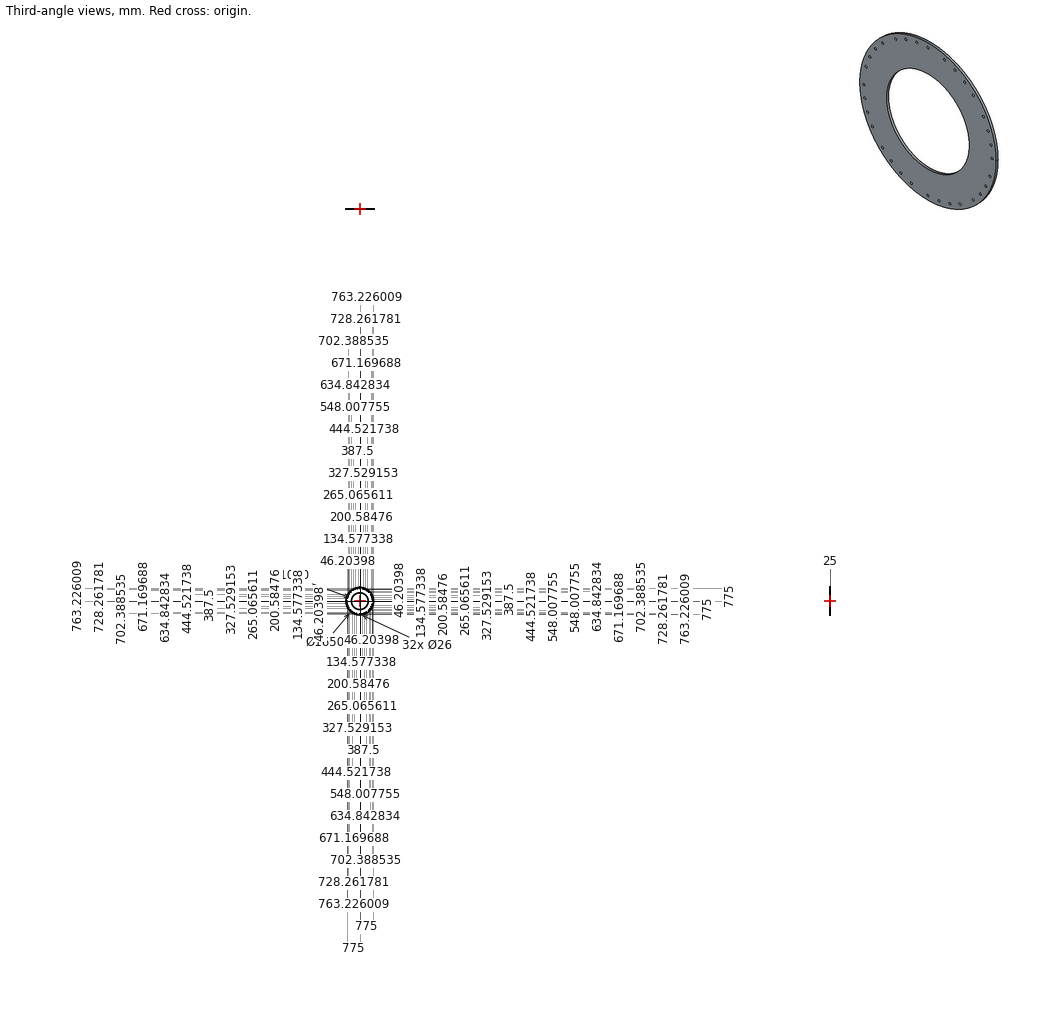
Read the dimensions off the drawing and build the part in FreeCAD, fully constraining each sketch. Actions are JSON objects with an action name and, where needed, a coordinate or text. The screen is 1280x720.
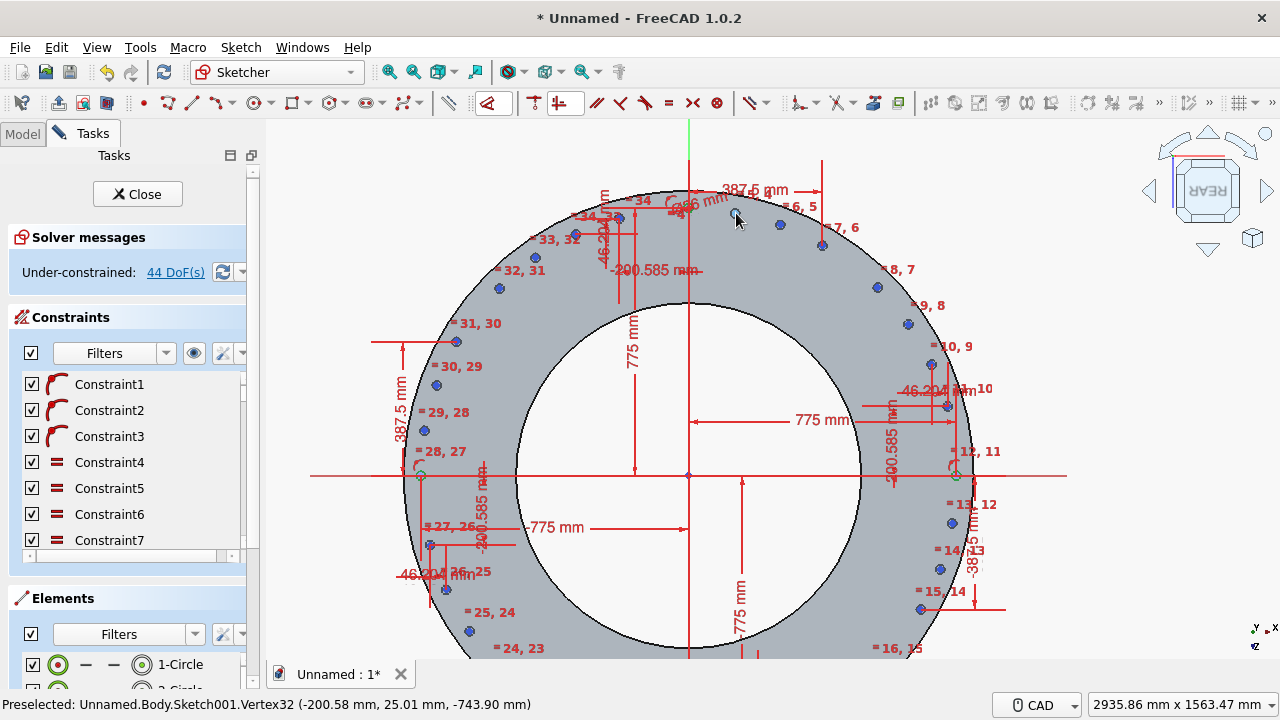
{"action": "left_click", "coordinate": [735, 213]}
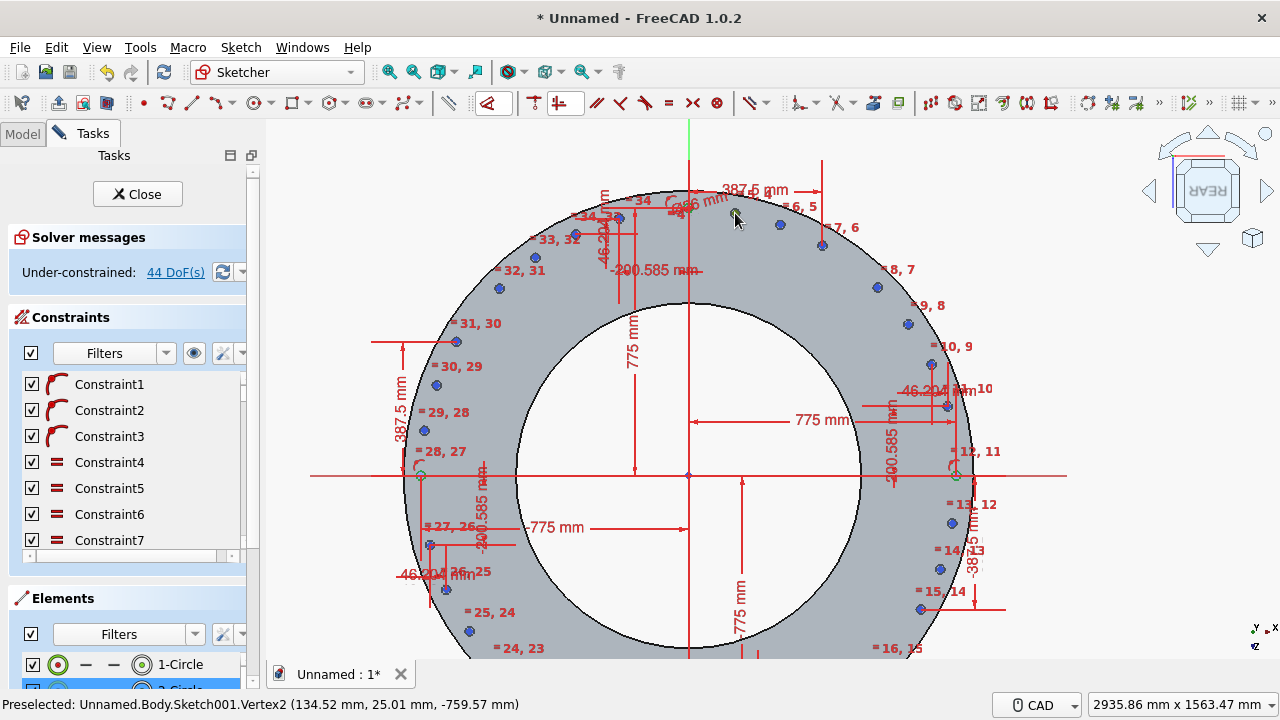
{"action": "left_click", "coordinate": [506, 104]}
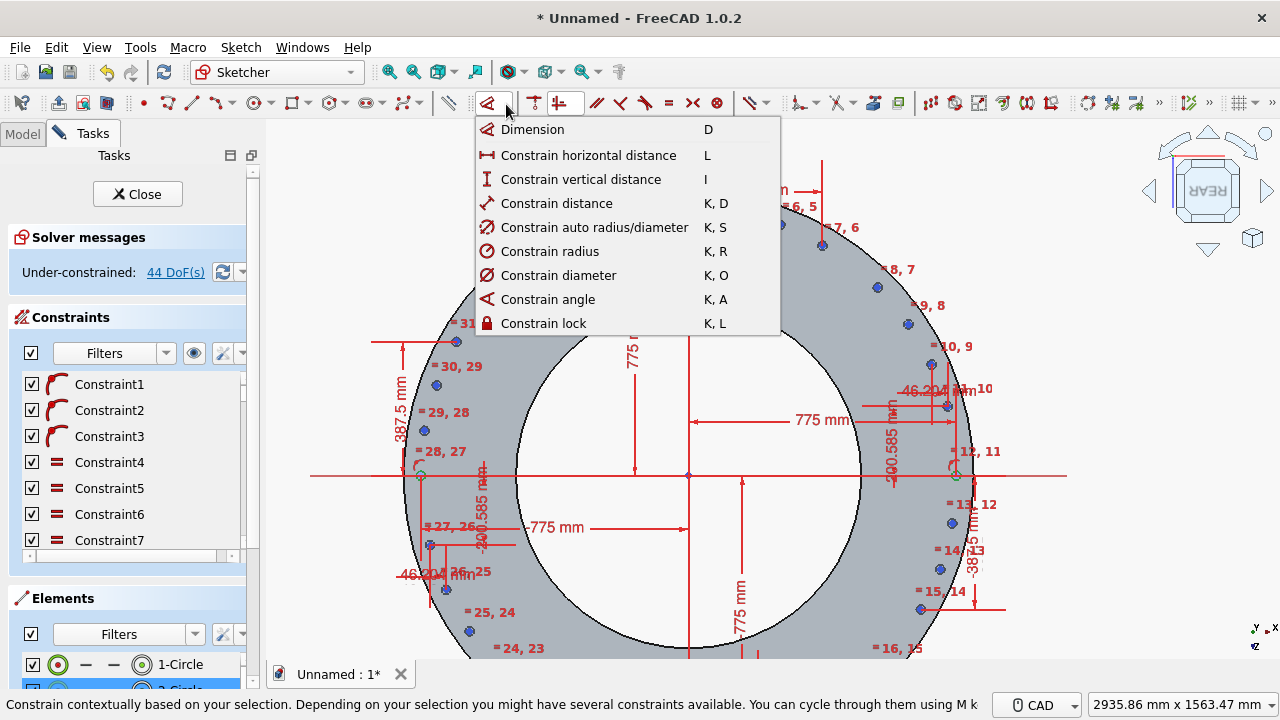
{"action": "left_click", "coordinate": [628, 155]}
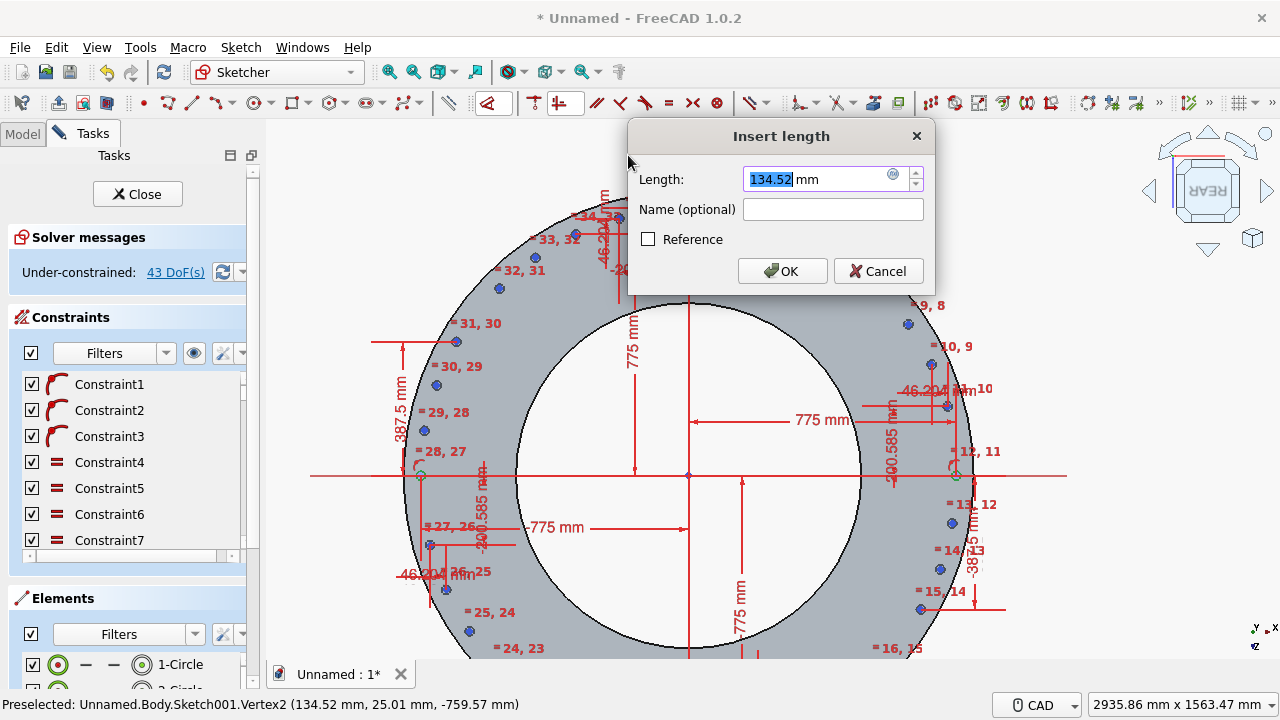
{"action": "type", "text": "134.577338"}
{"action": "key", "text": "Return"}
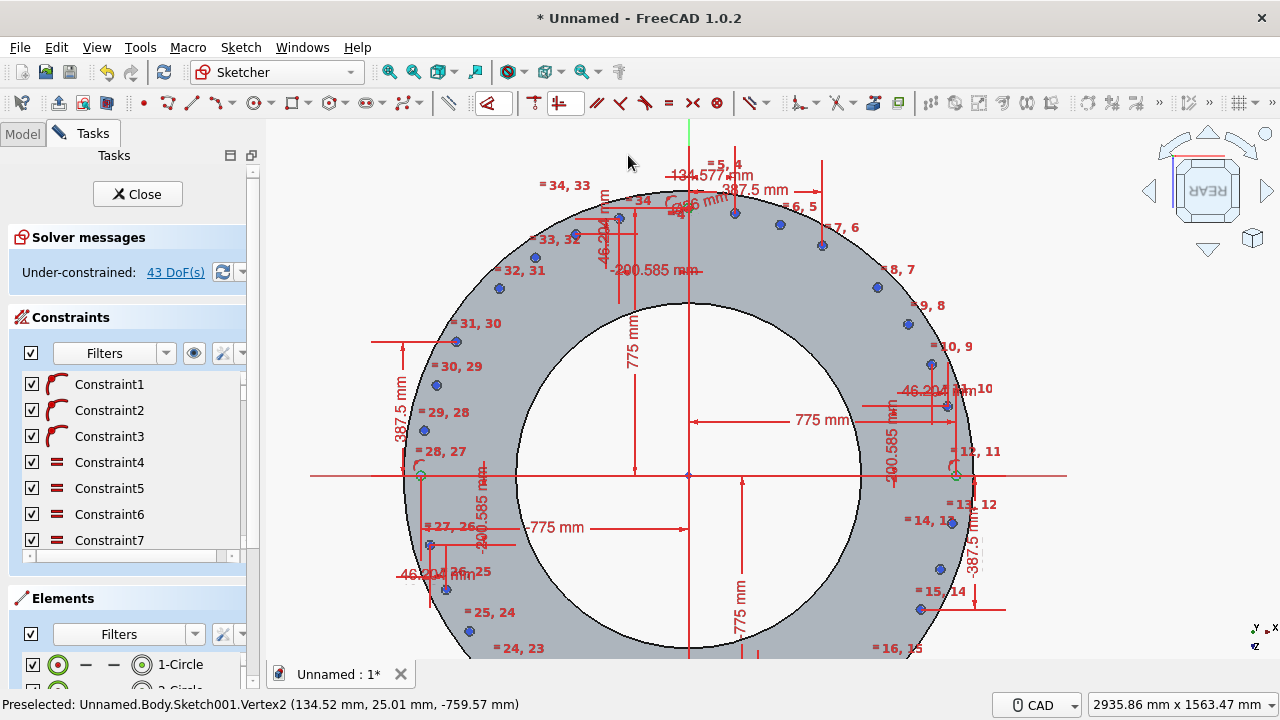
{"action": "left_click", "coordinate": [735, 213]}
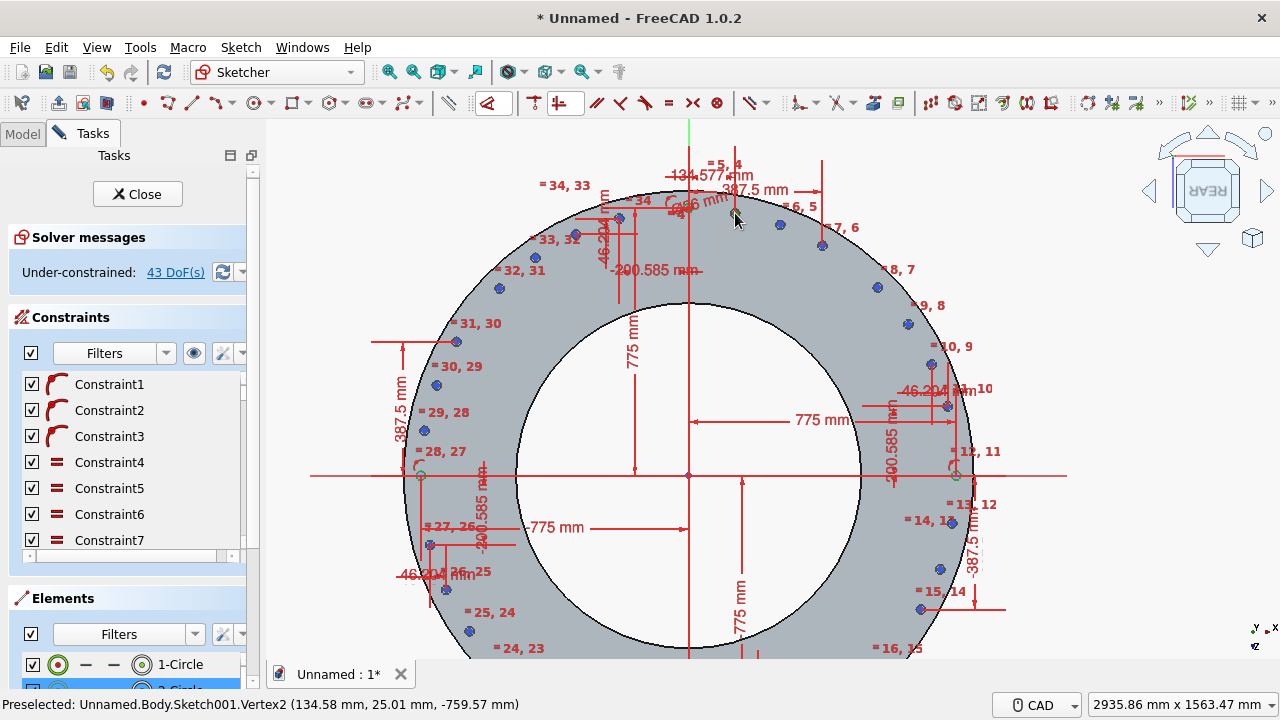
{"action": "key", "text": "i"}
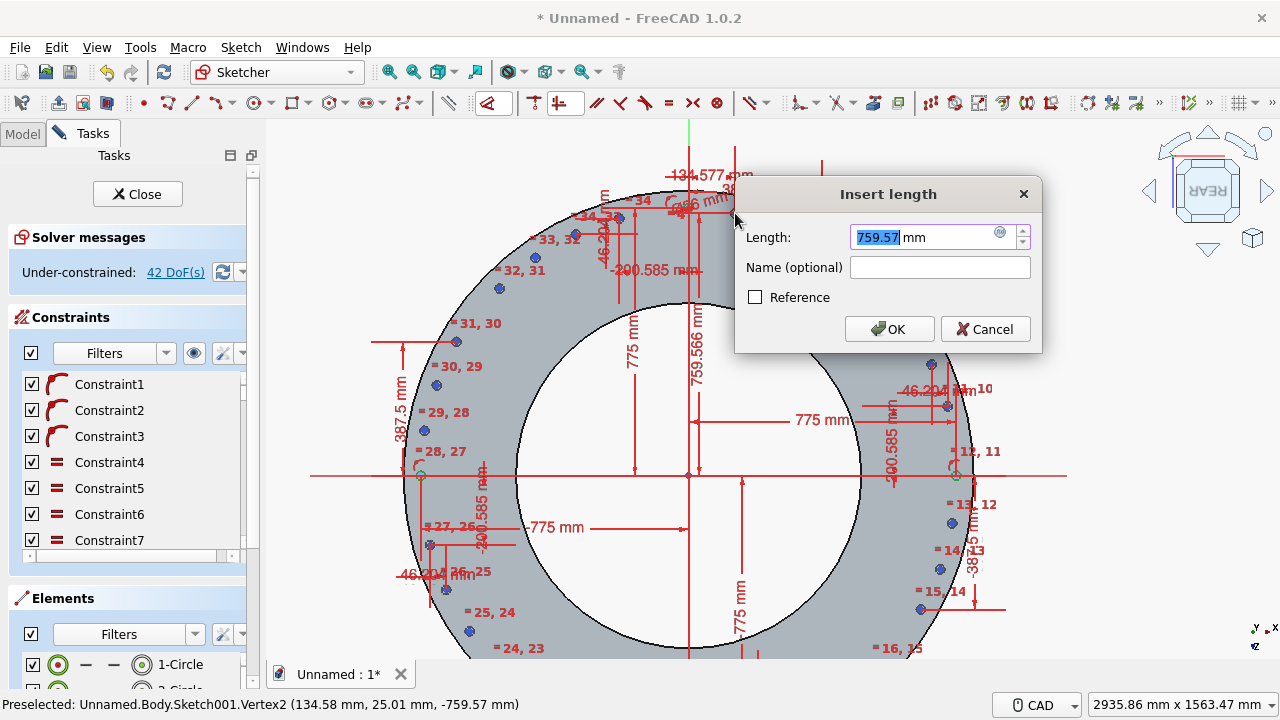
{"action": "type", "text": "763.226009"}
{"action": "key", "text": "Return"}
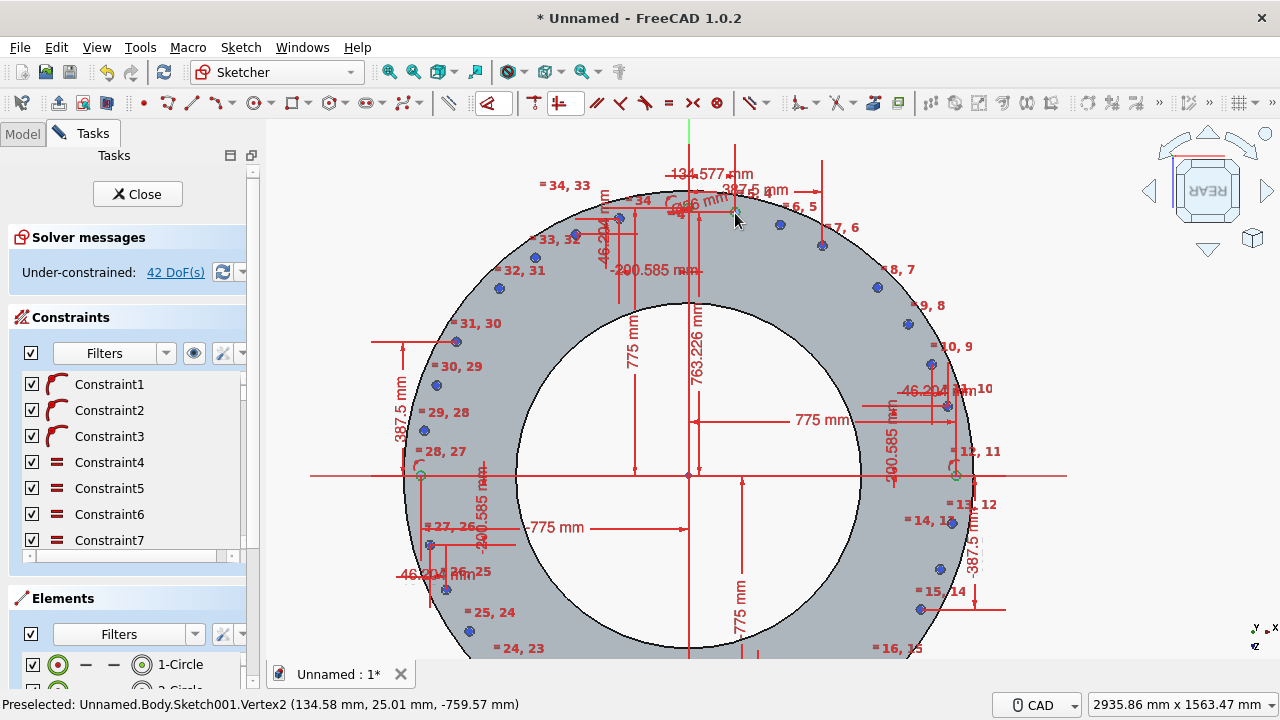
{"action": "left_click", "coordinate": [780, 225]}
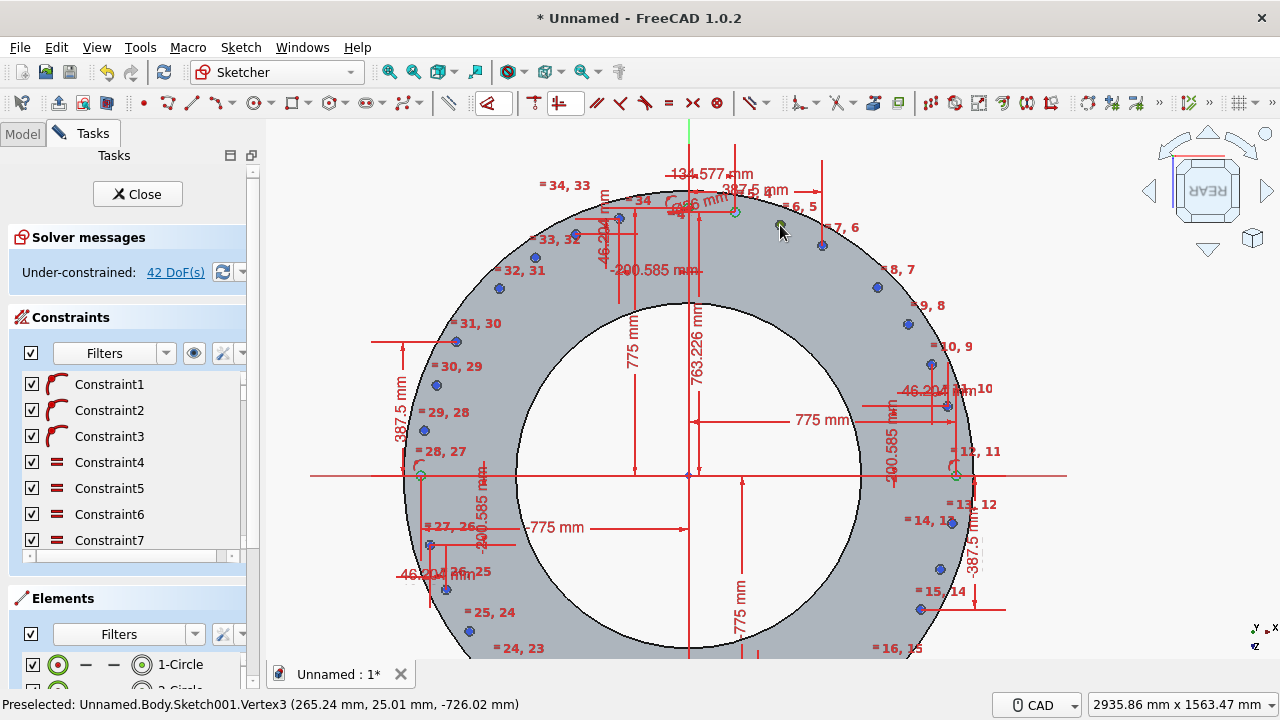
{"action": "left_click", "coordinate": [506, 104]}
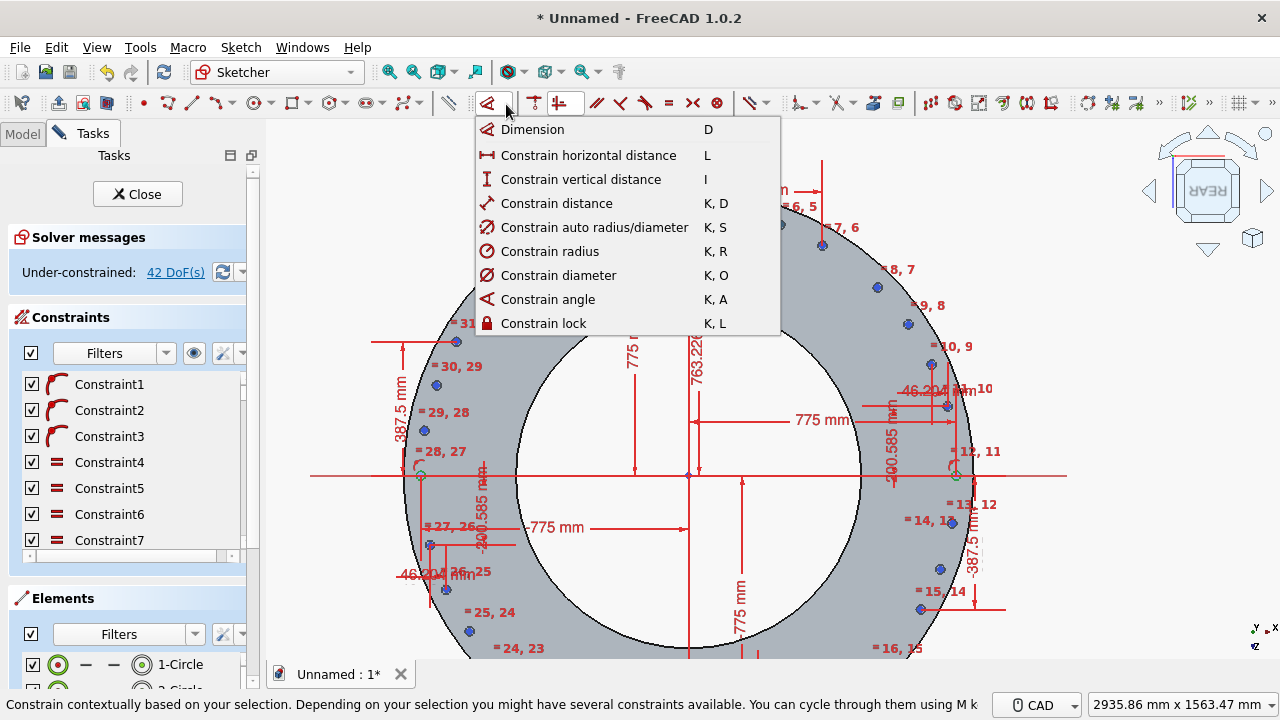
{"action": "left_click", "coordinate": [628, 155]}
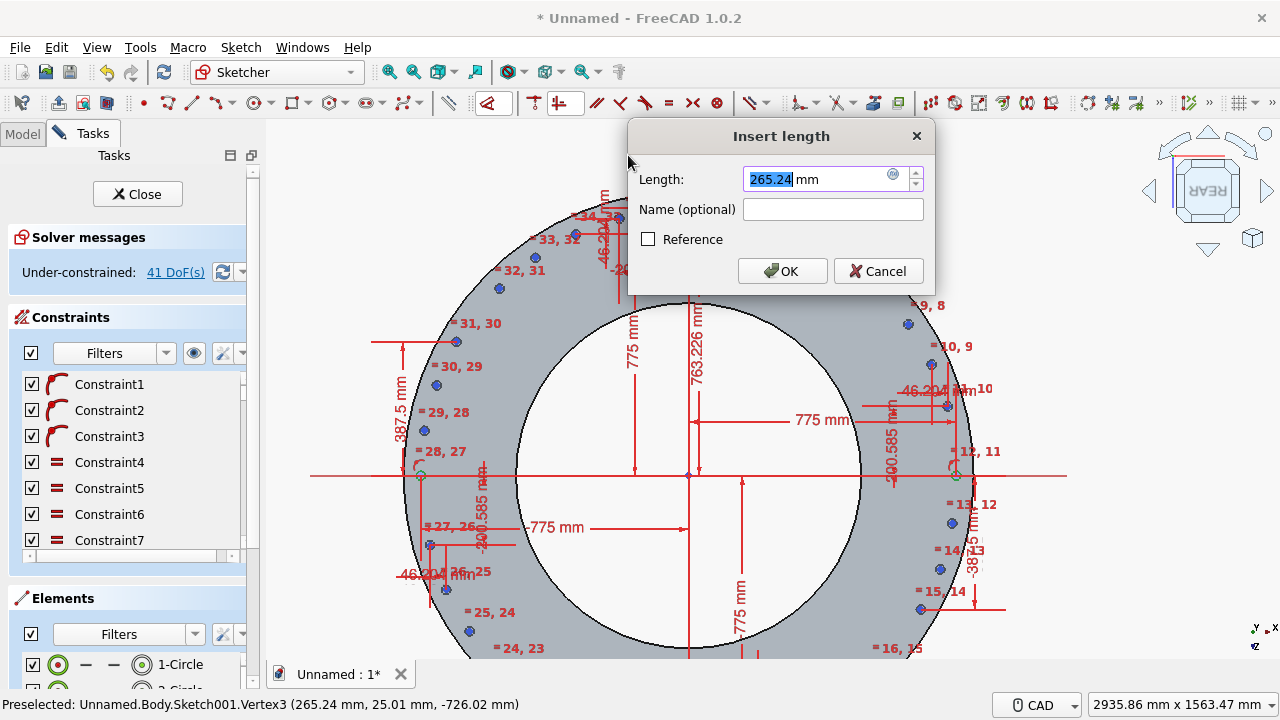
{"action": "type", "text": "265.065611"}
{"action": "key", "text": "Return"}